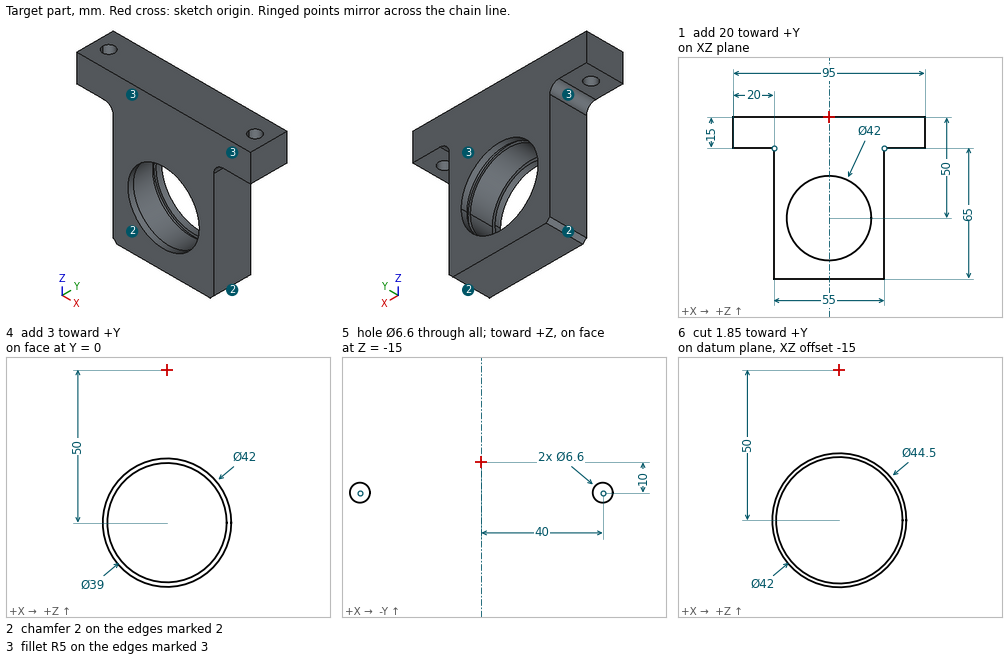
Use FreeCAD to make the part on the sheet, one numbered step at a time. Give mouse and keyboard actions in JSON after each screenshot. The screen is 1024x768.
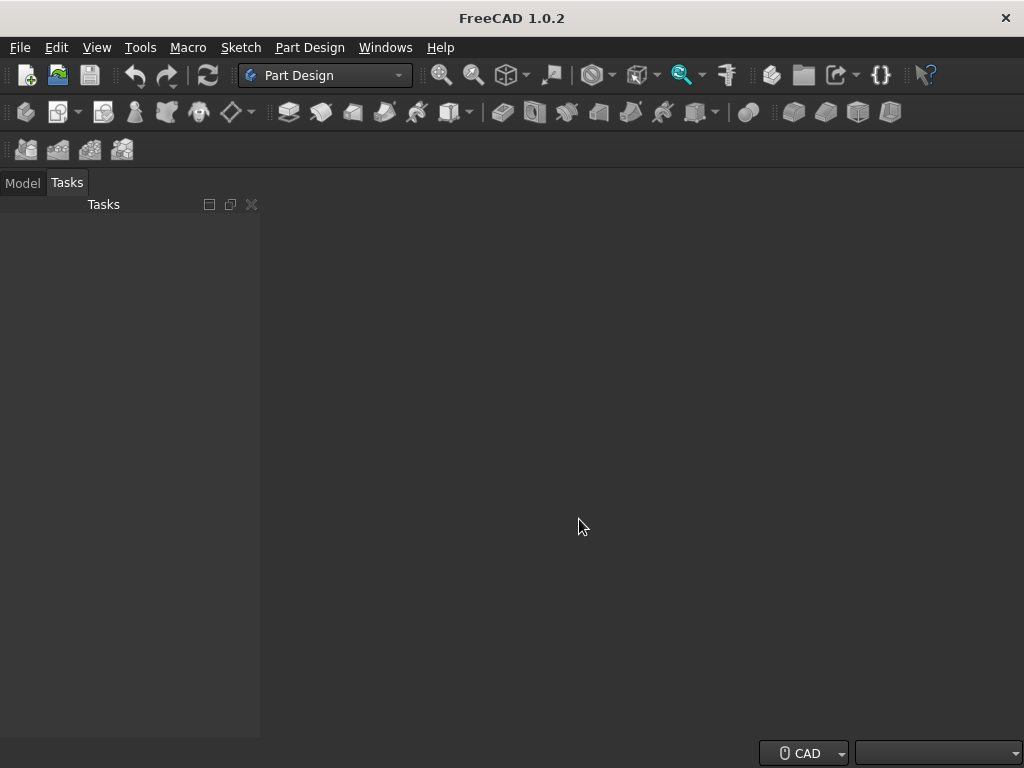
{"action": "left_click", "coordinate": [26, 76]}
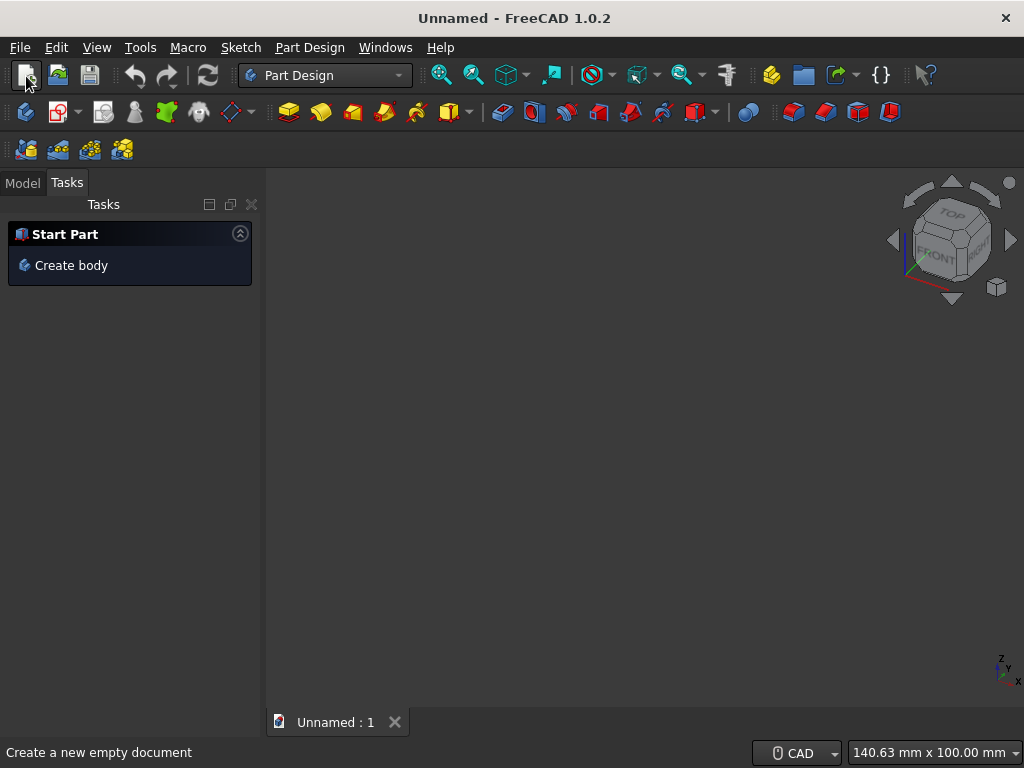
{"action": "left_click", "coordinate": [58, 112]}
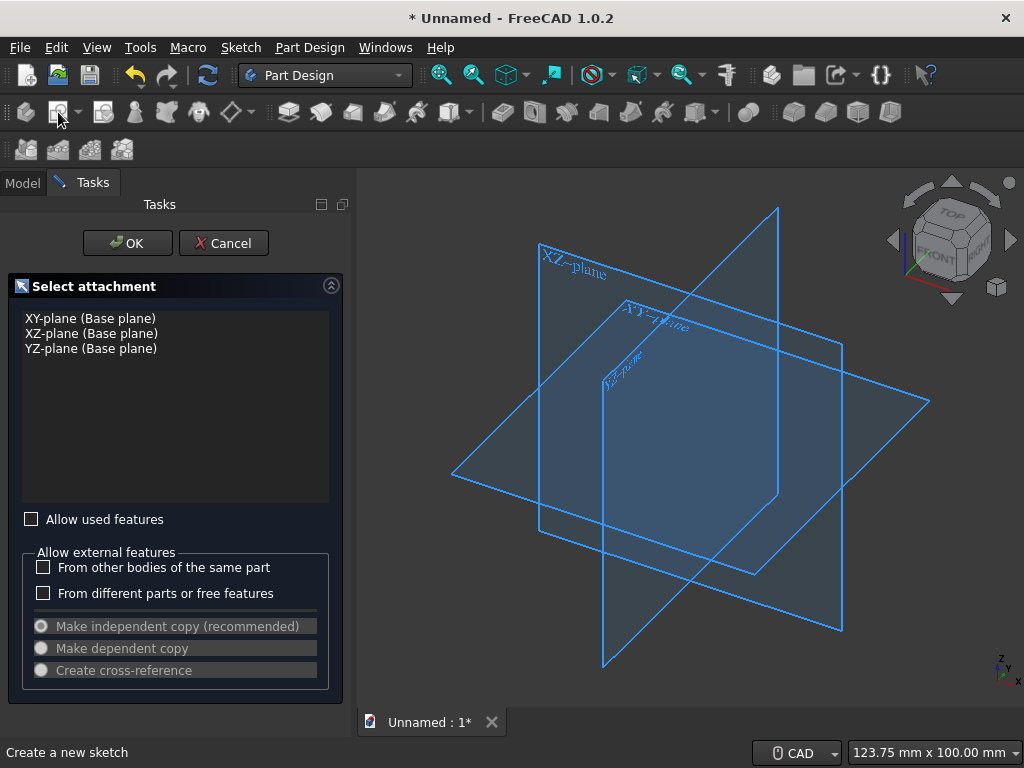
{"action": "left_click", "coordinate": [82, 334]}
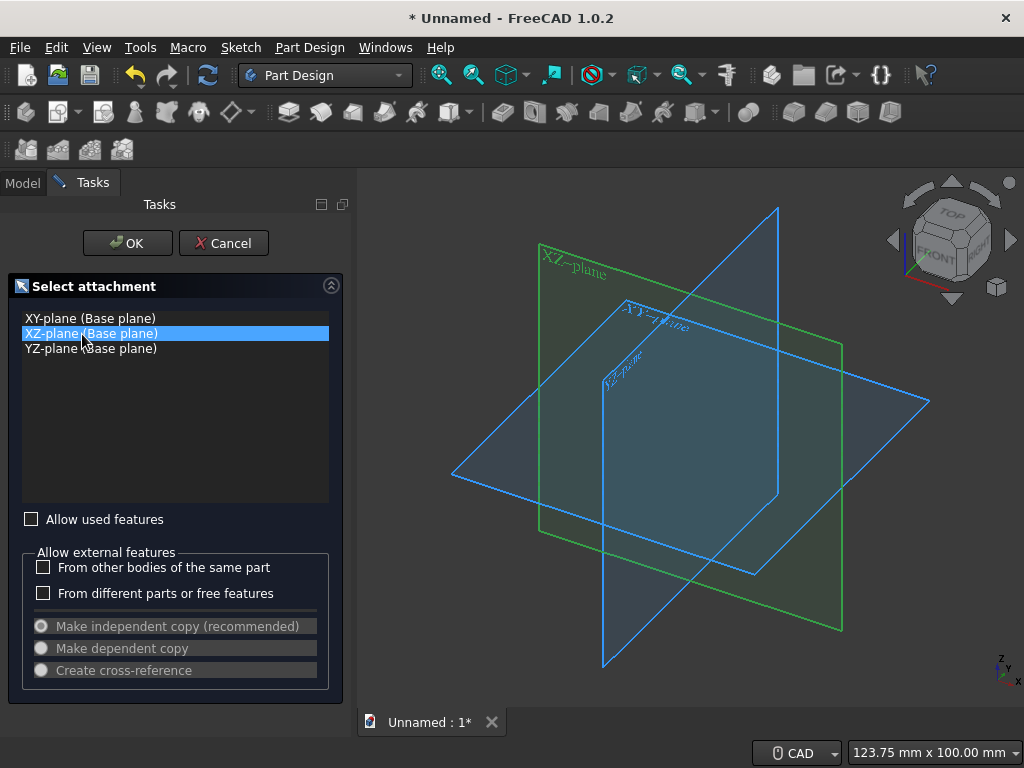
{"action": "left_click", "coordinate": [128, 243]}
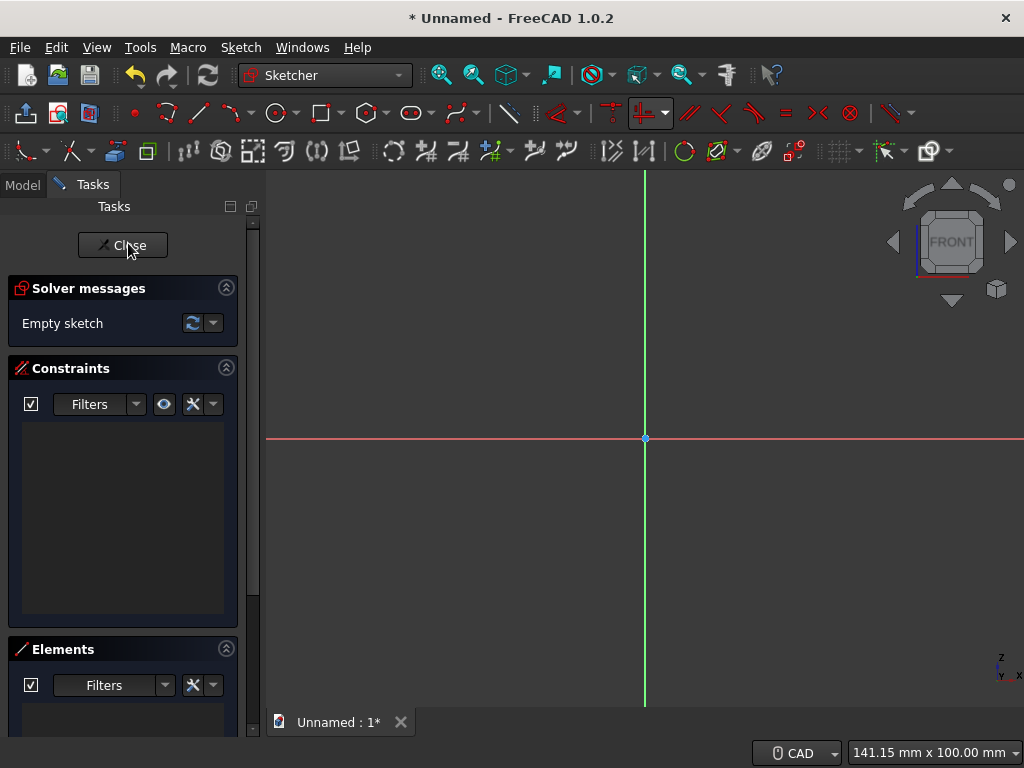
{"action": "scroll", "coordinate": [437, 198], "scroll_direction": "down", "scroll_amount": 2}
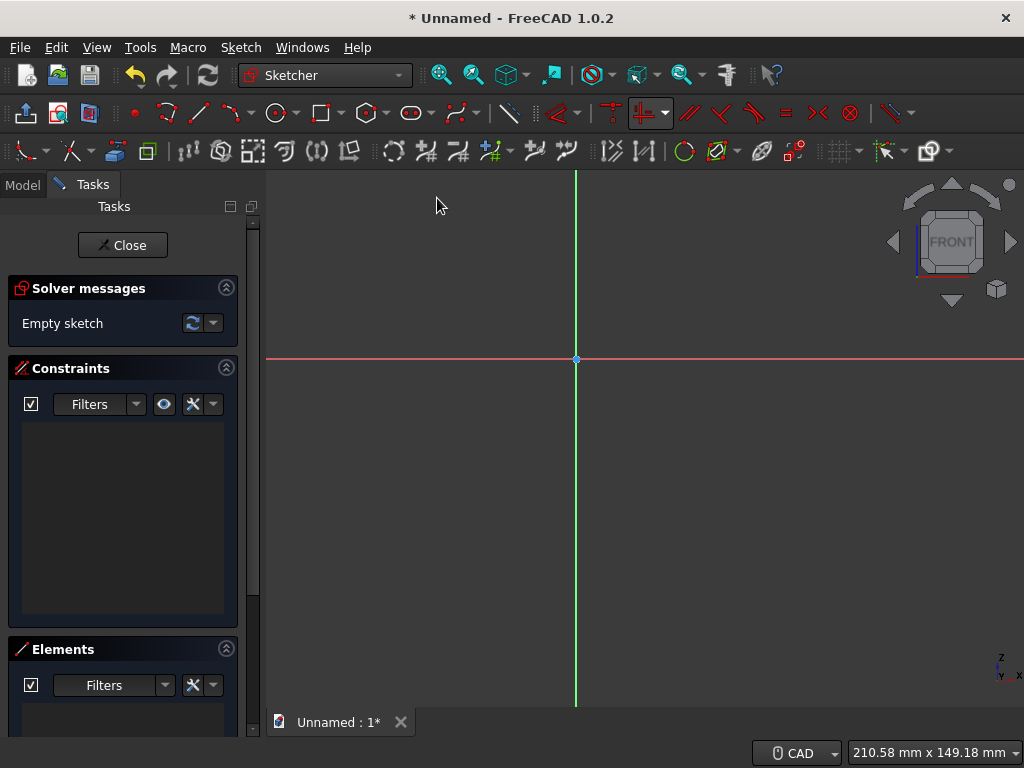
{"action": "key", "text": "g m"}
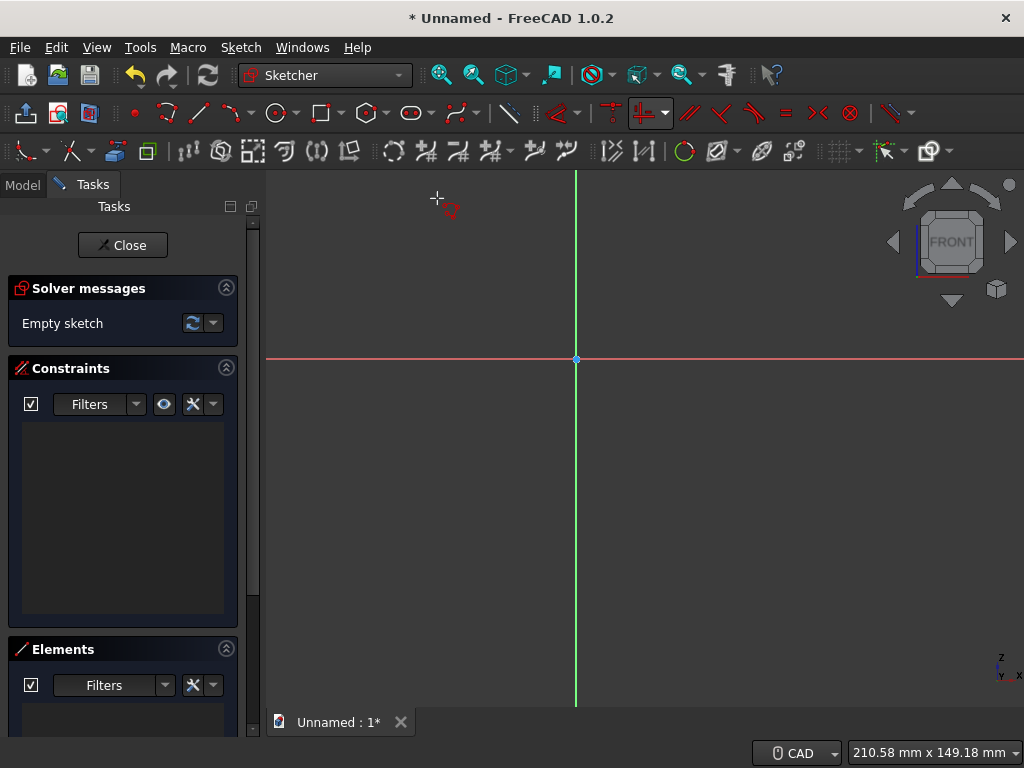
{"action": "left_click", "coordinate": [675, 413]}
{"action": "left_click", "coordinate": [675, 647]}
{"action": "left_click", "coordinate": [478, 647]}
{"action": "left_click", "coordinate": [478, 413]}
{"action": "left_click", "coordinate": [406, 413]}
{"action": "left_click", "coordinate": [406, 359]}
{"action": "left_click", "coordinate": [747, 368]}
{"action": "left_click", "coordinate": [747, 413]}
{"action": "left_click", "coordinate": [675, 414]}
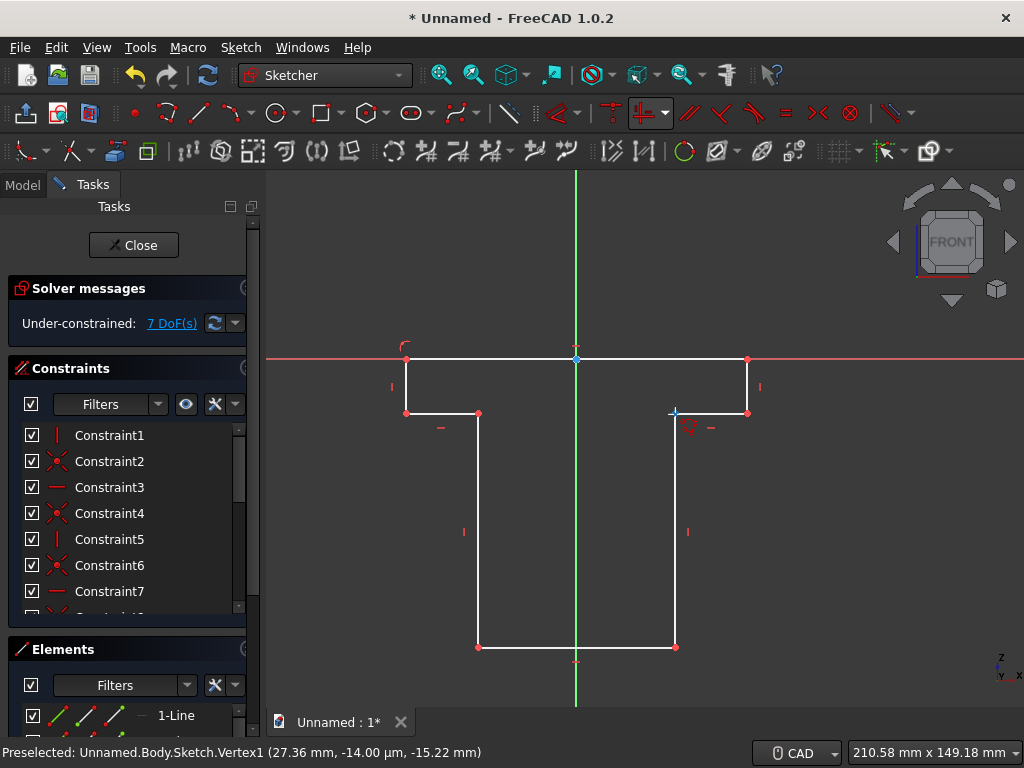
{"action": "left_click", "coordinate": [276, 114]}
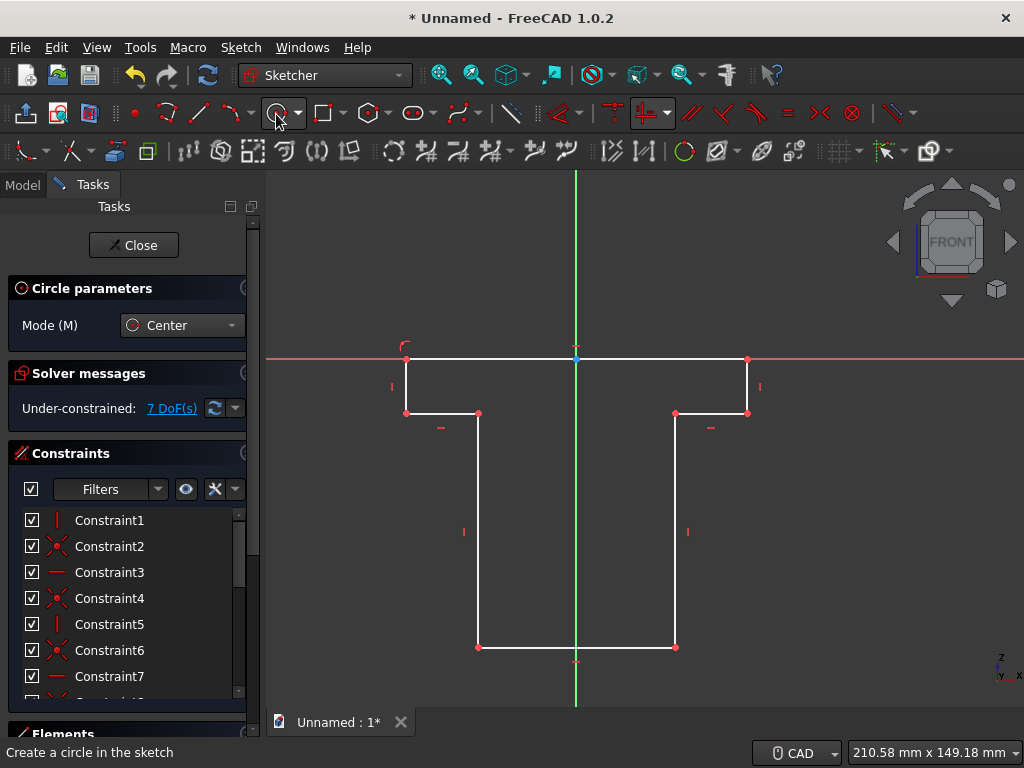
{"action": "left_click", "coordinate": [577, 539]}
{"action": "mouse_move", "coordinate": [630, 486]}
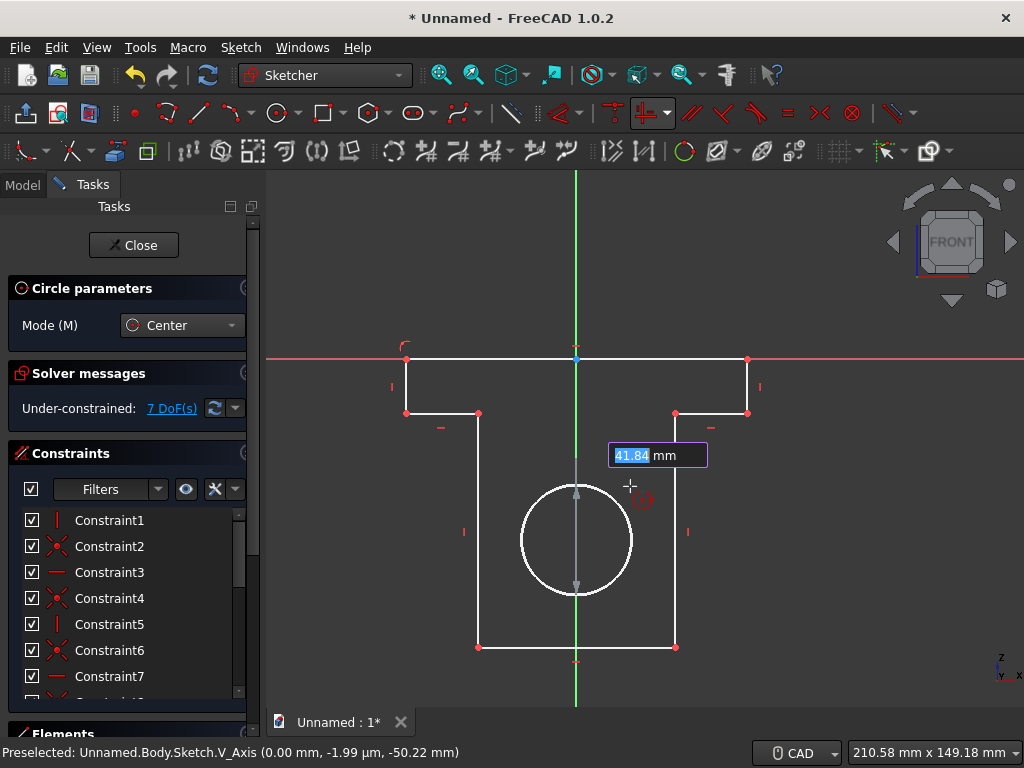
{"action": "type", "text": "42"}
{"action": "key", "text": "Return"}
{"action": "key", "text": "Escape"}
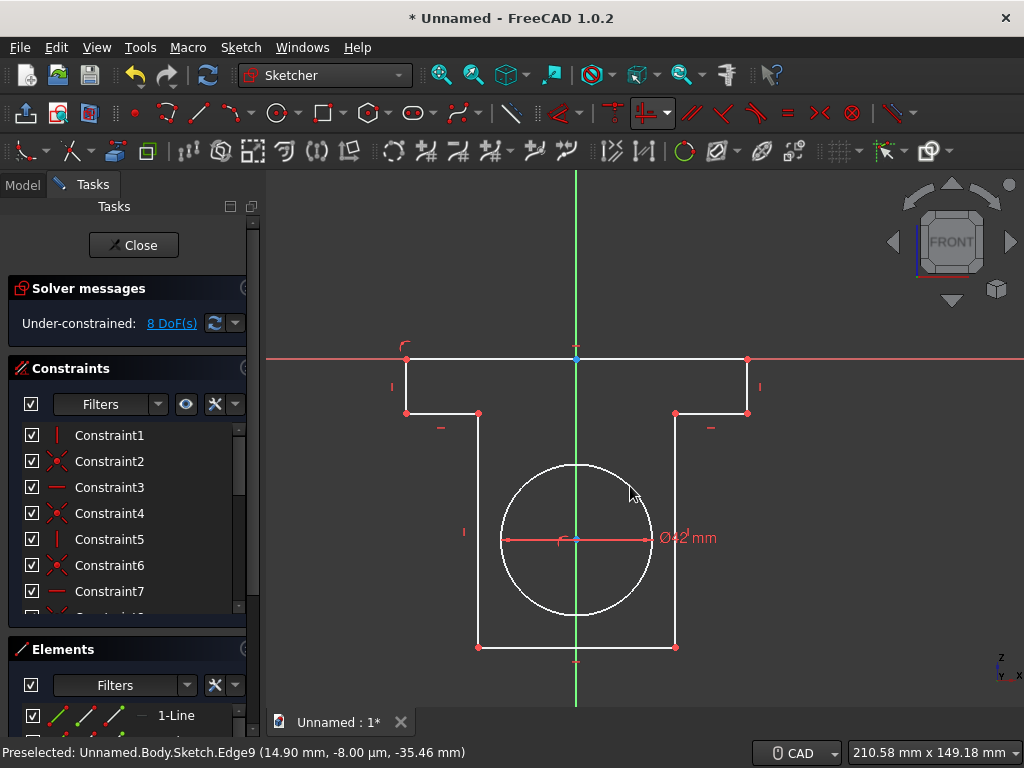
{"action": "left_click", "coordinate": [675, 414]}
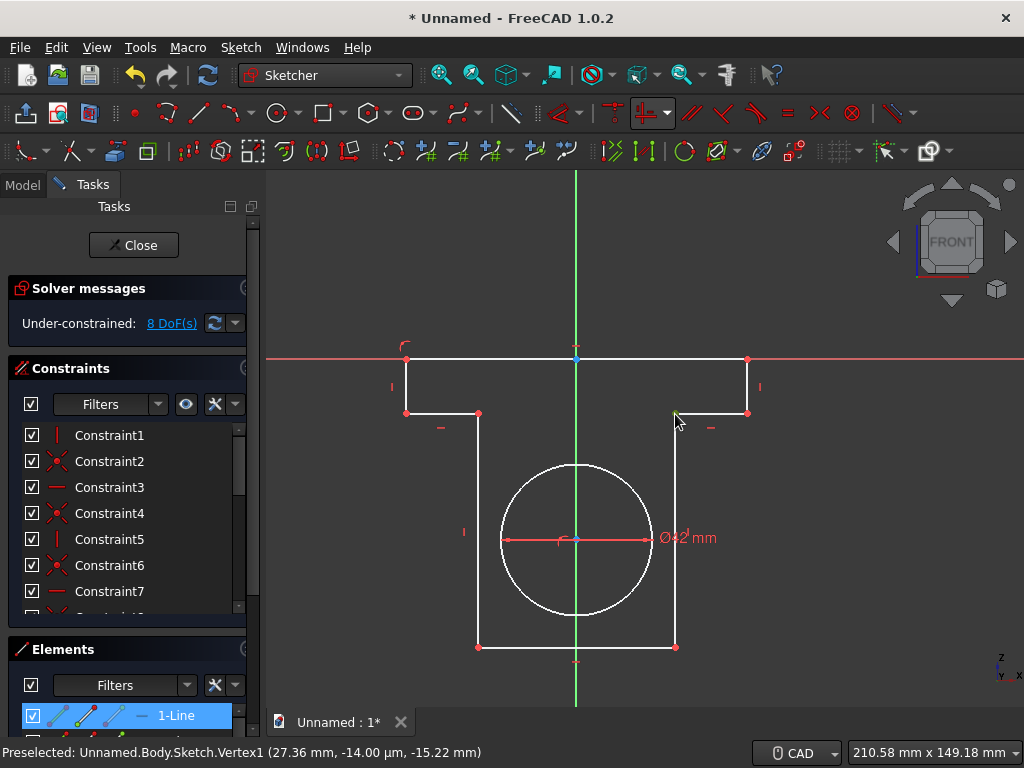
{"action": "left_click", "coordinate": [478, 414]}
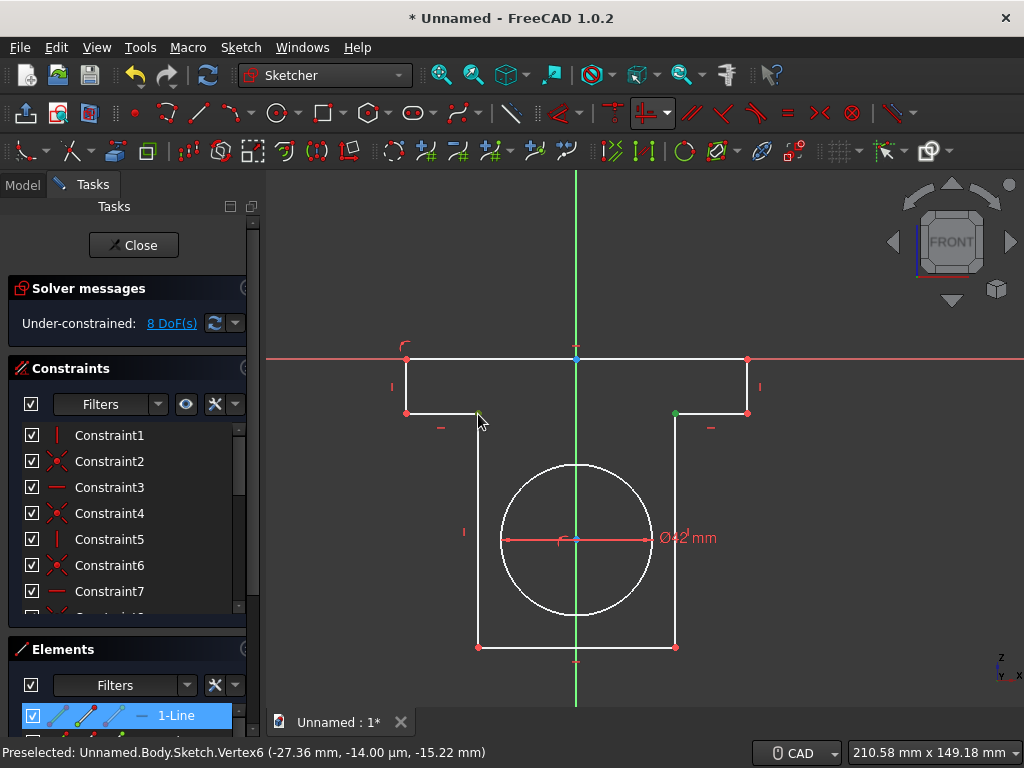
{"action": "left_click", "coordinate": [577, 576]}